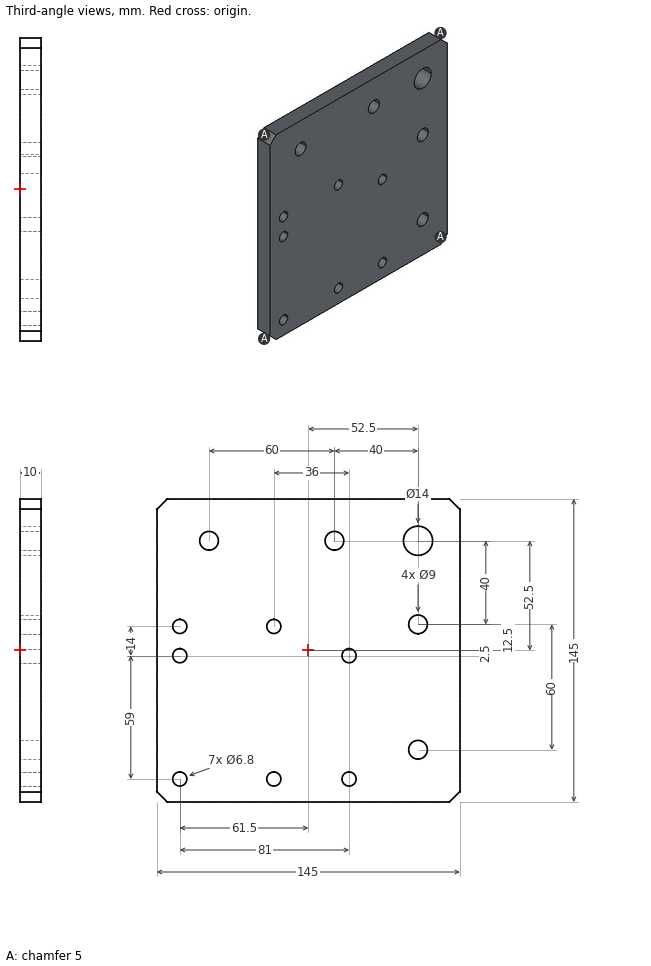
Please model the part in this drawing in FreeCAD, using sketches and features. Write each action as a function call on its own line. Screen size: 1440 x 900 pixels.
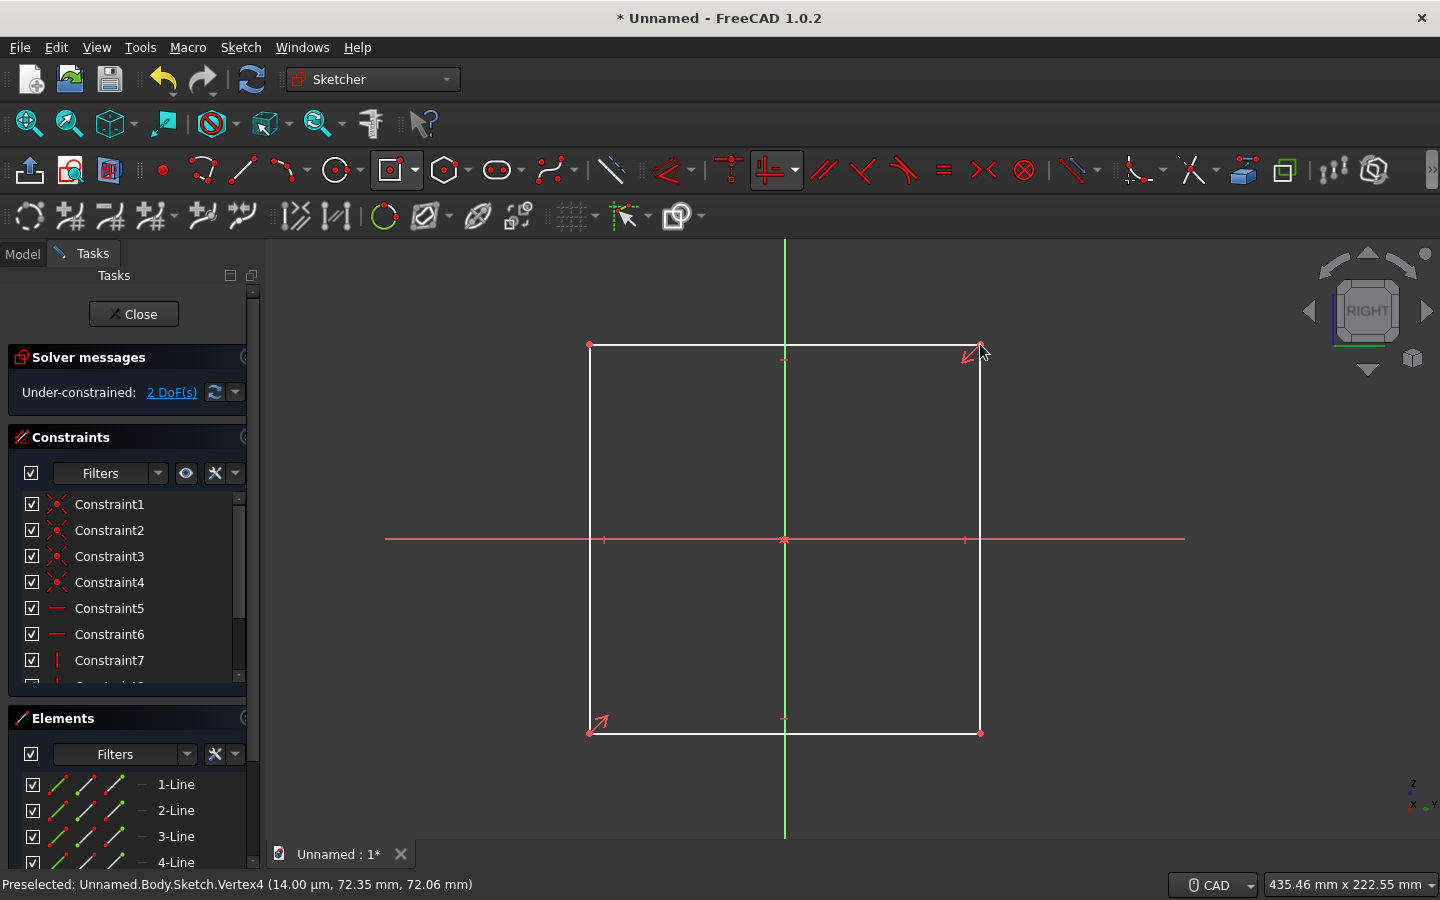
click(666, 170)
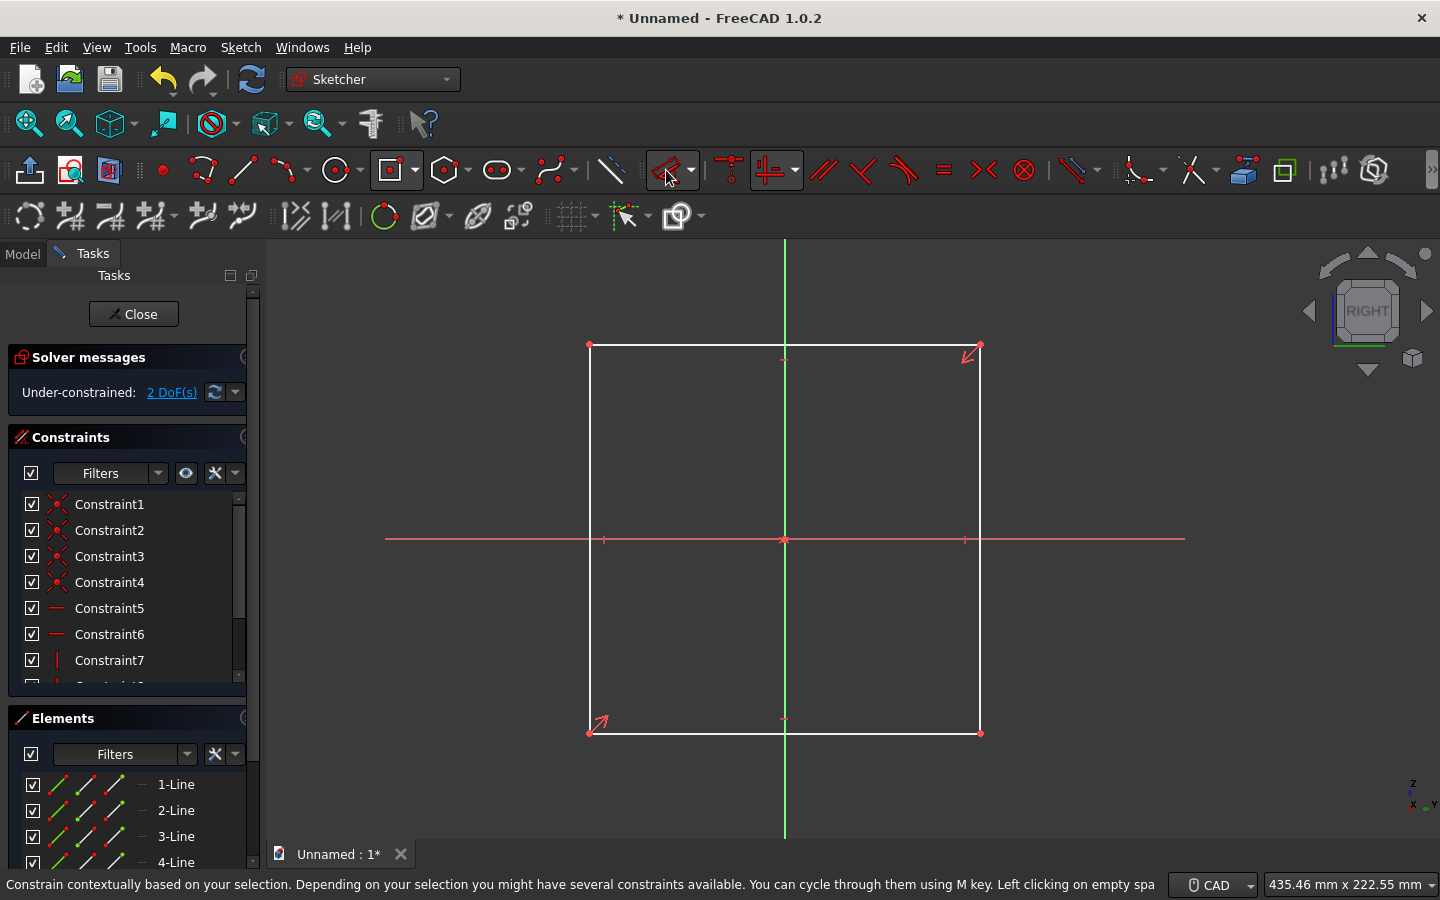
click(707, 734)
click(695, 768)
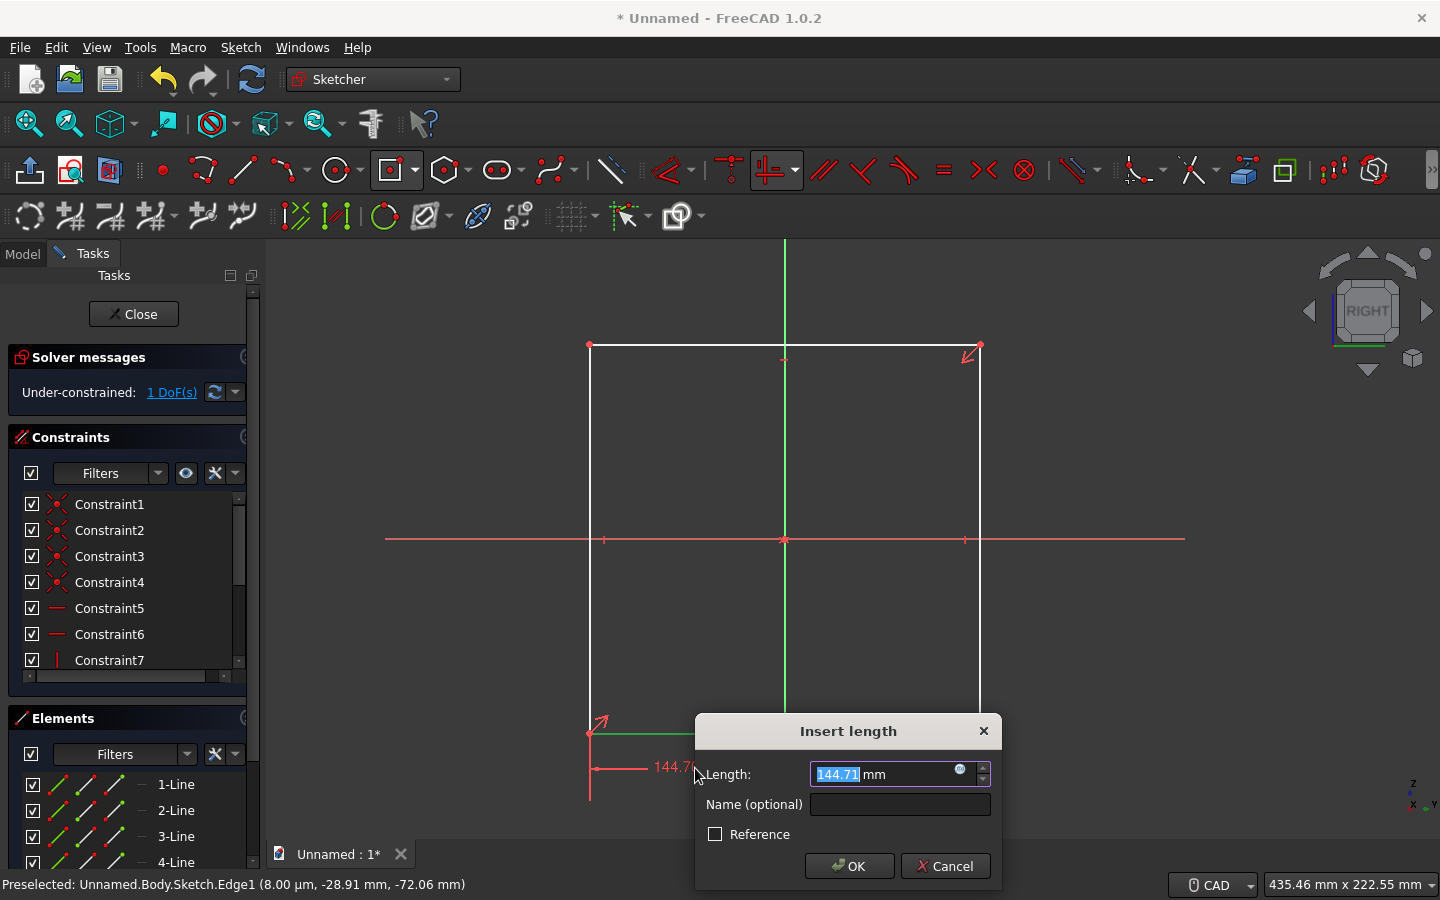
text(145)
key(Return)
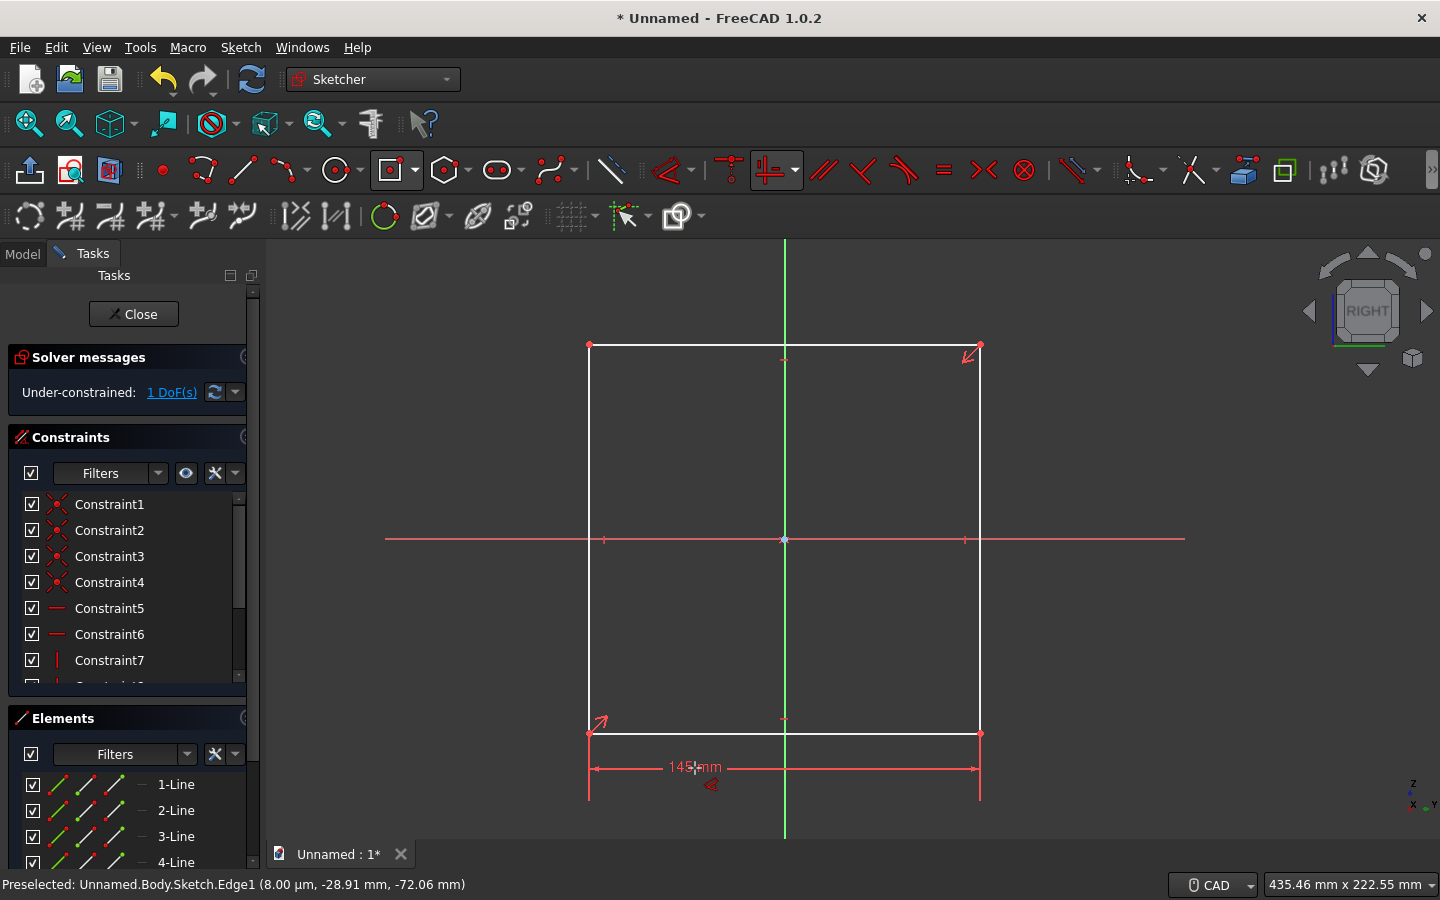
click(980, 617)
click(1014, 450)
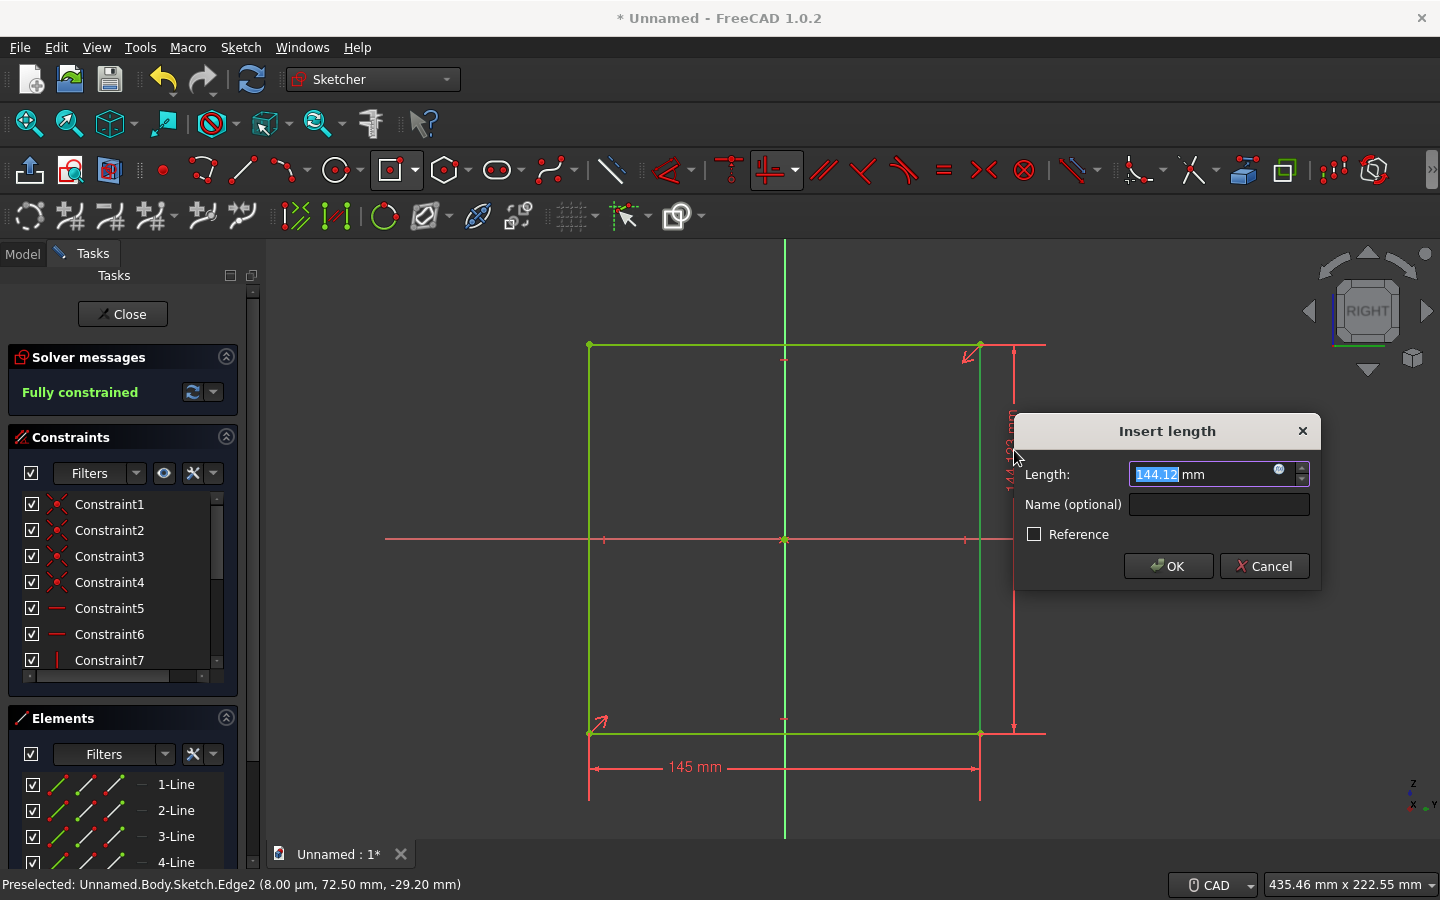
text(145)
key(Return)
key(Escape)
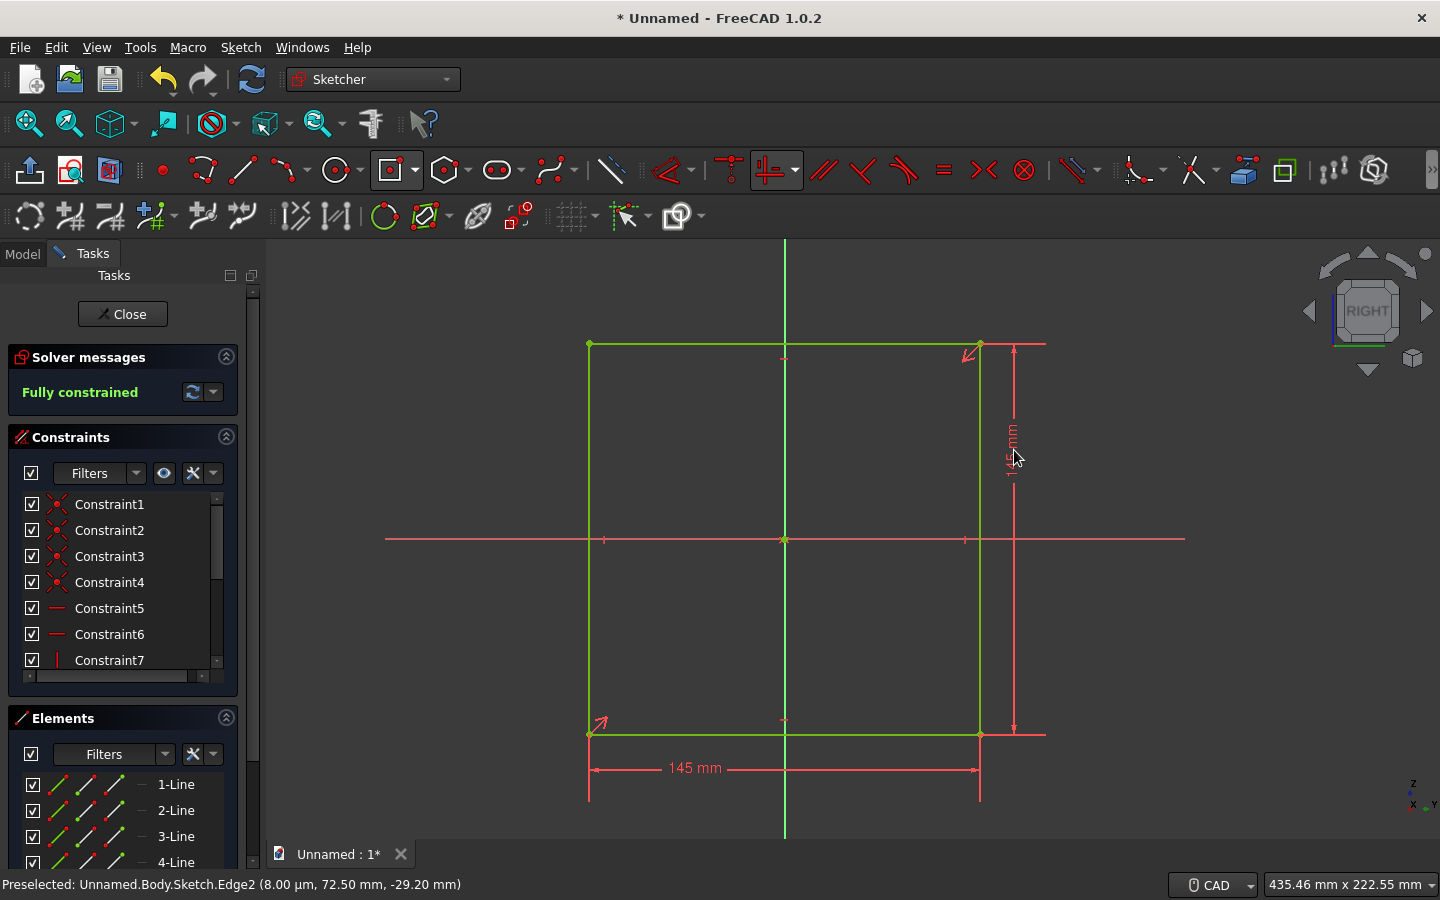
click(123, 314)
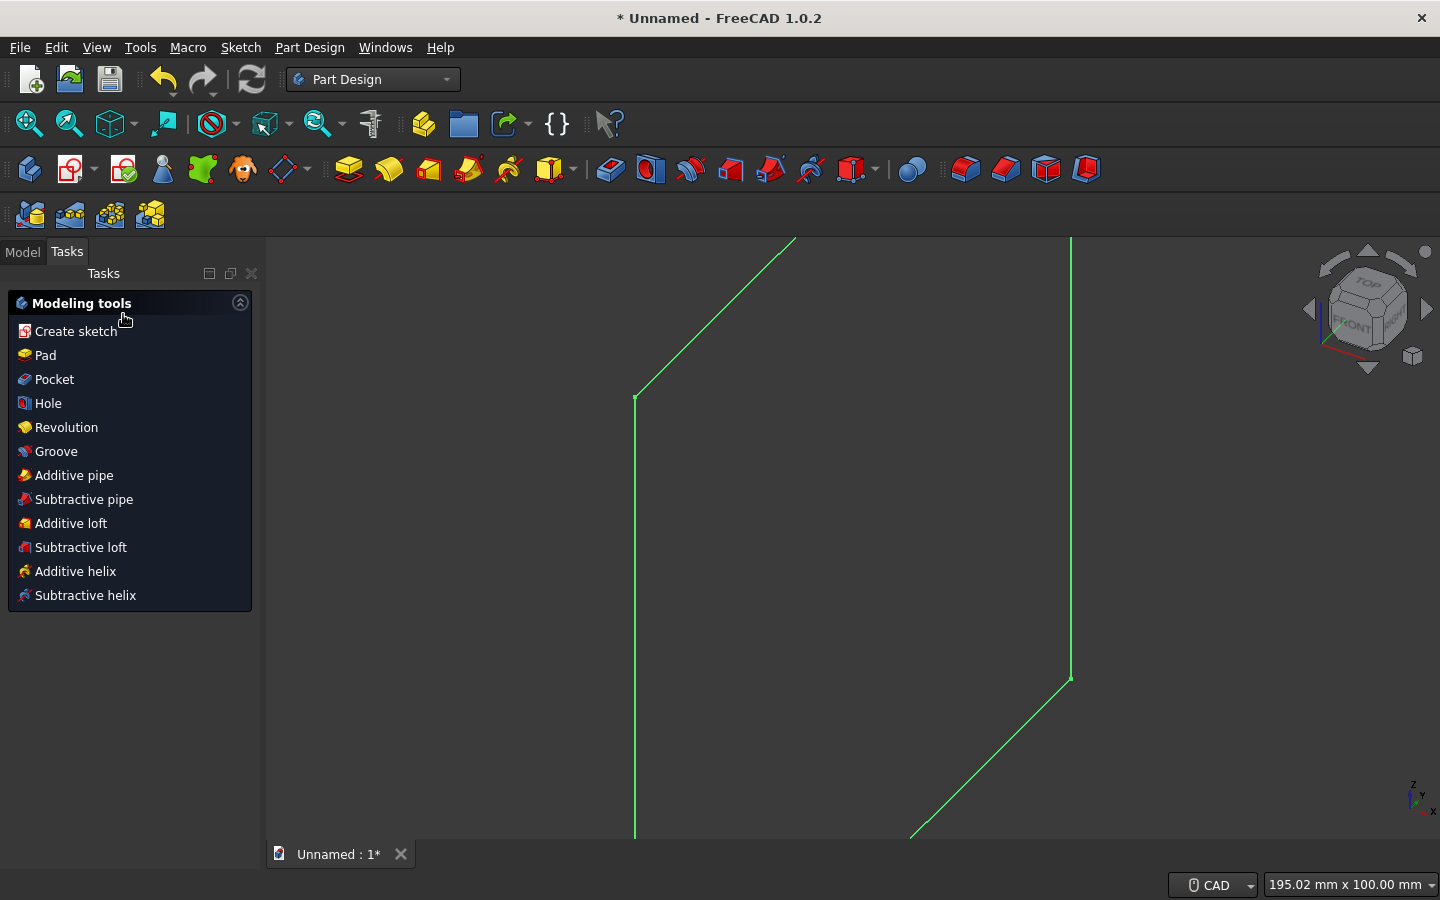
click(350, 170)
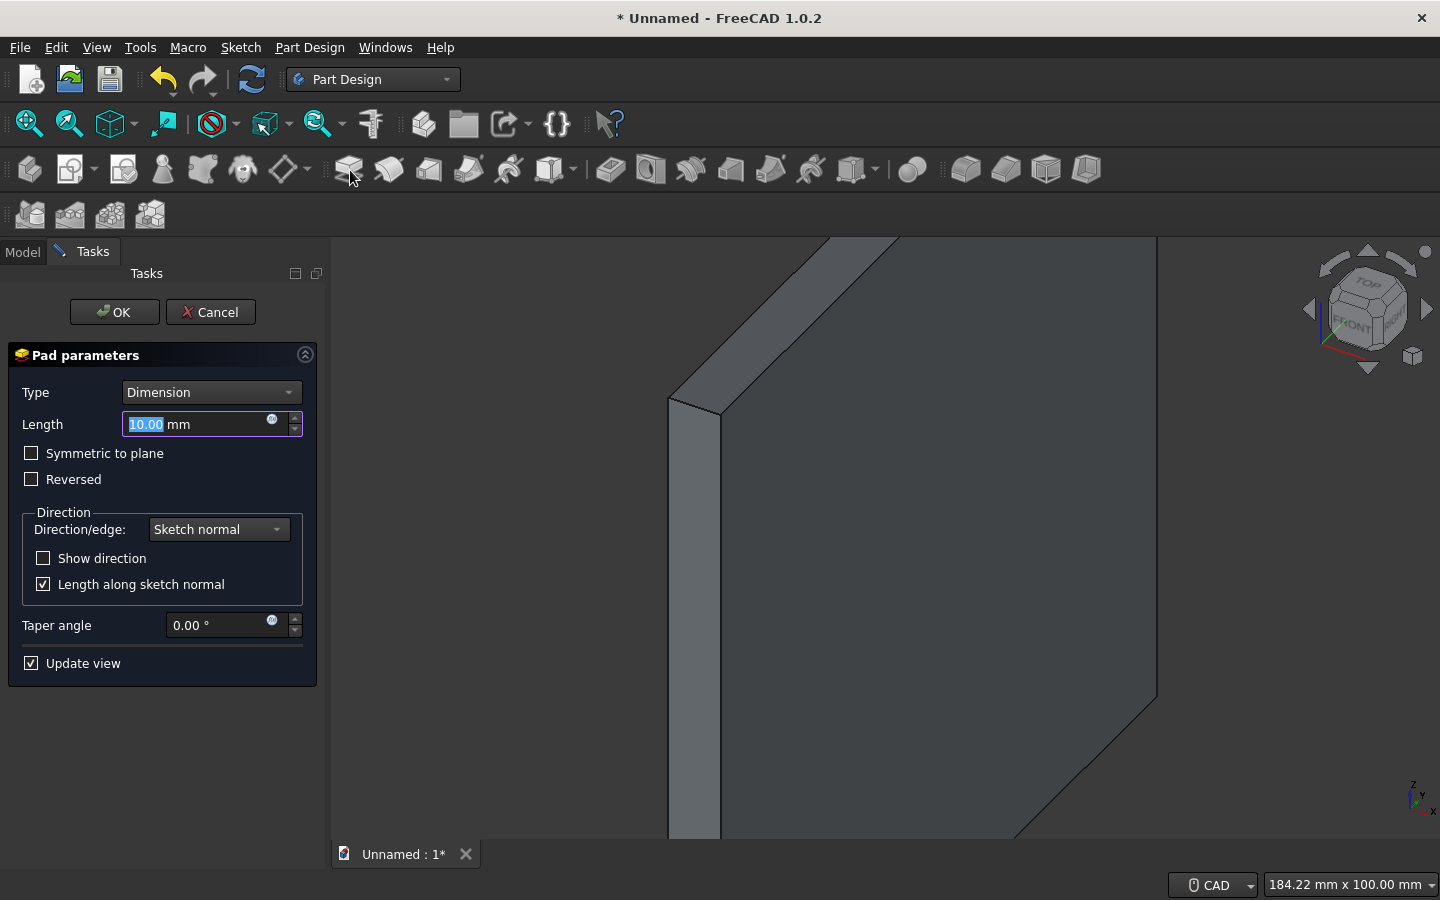
text(10)
key(Tab)